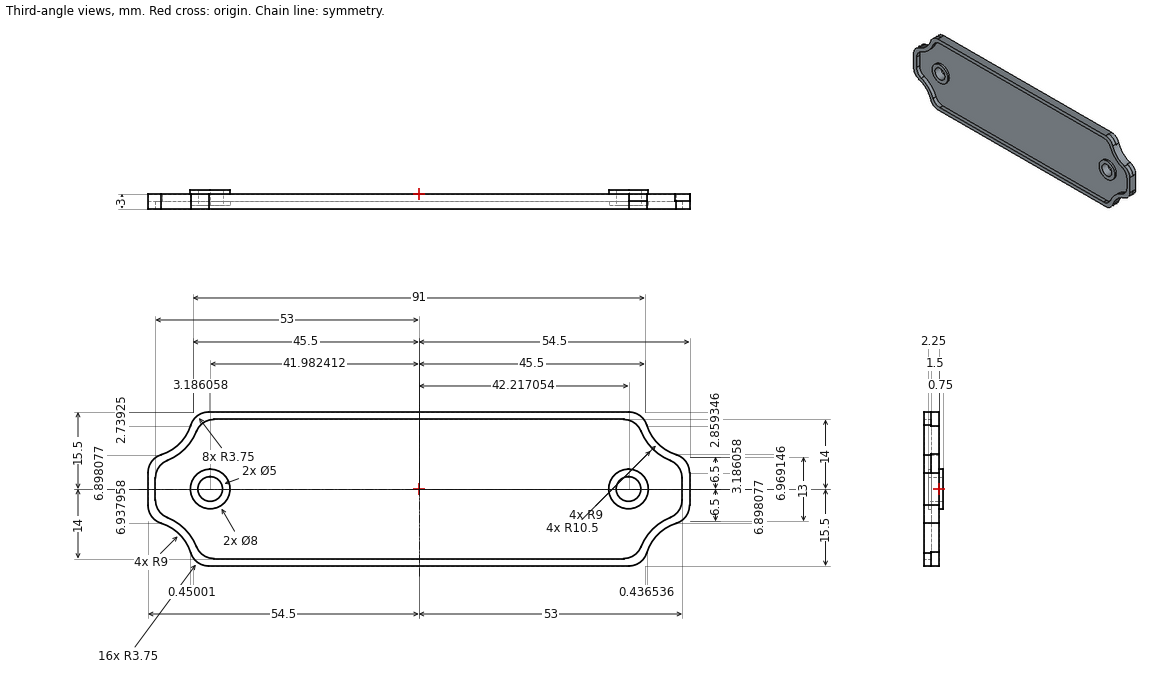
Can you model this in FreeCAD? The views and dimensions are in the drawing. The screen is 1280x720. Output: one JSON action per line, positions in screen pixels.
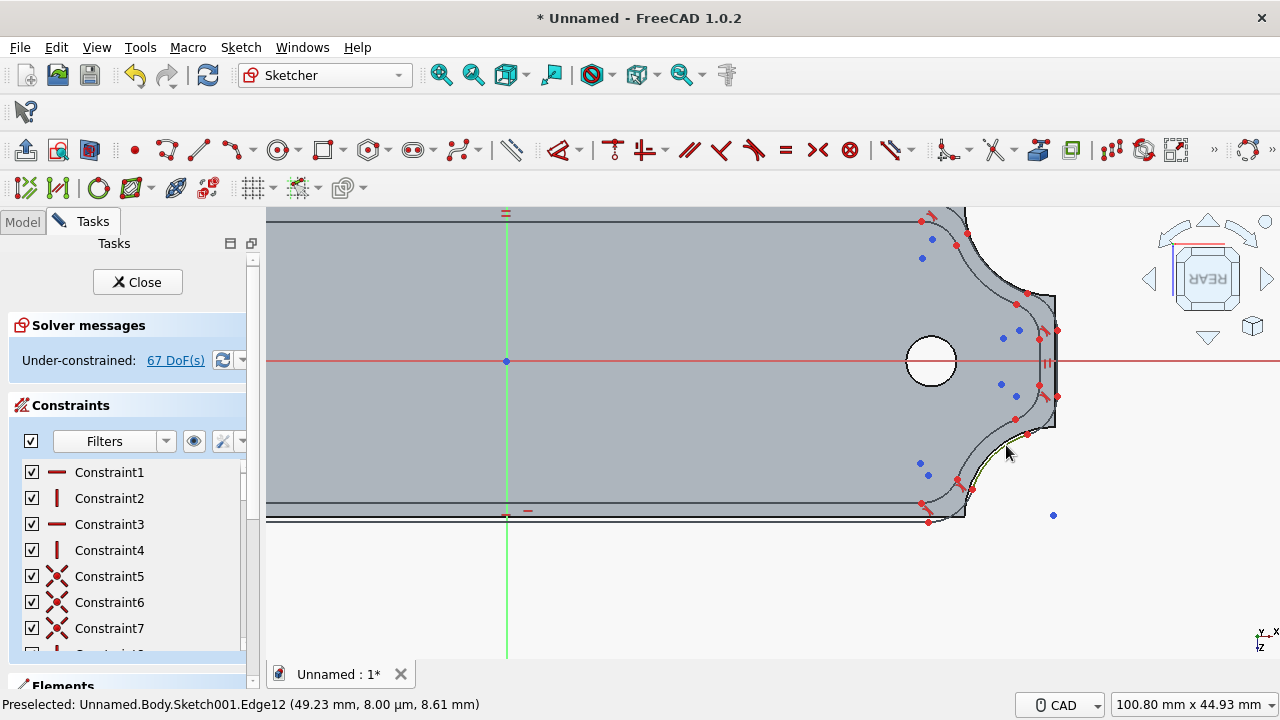
{"action": "left_click", "coordinate": [1042, 428]}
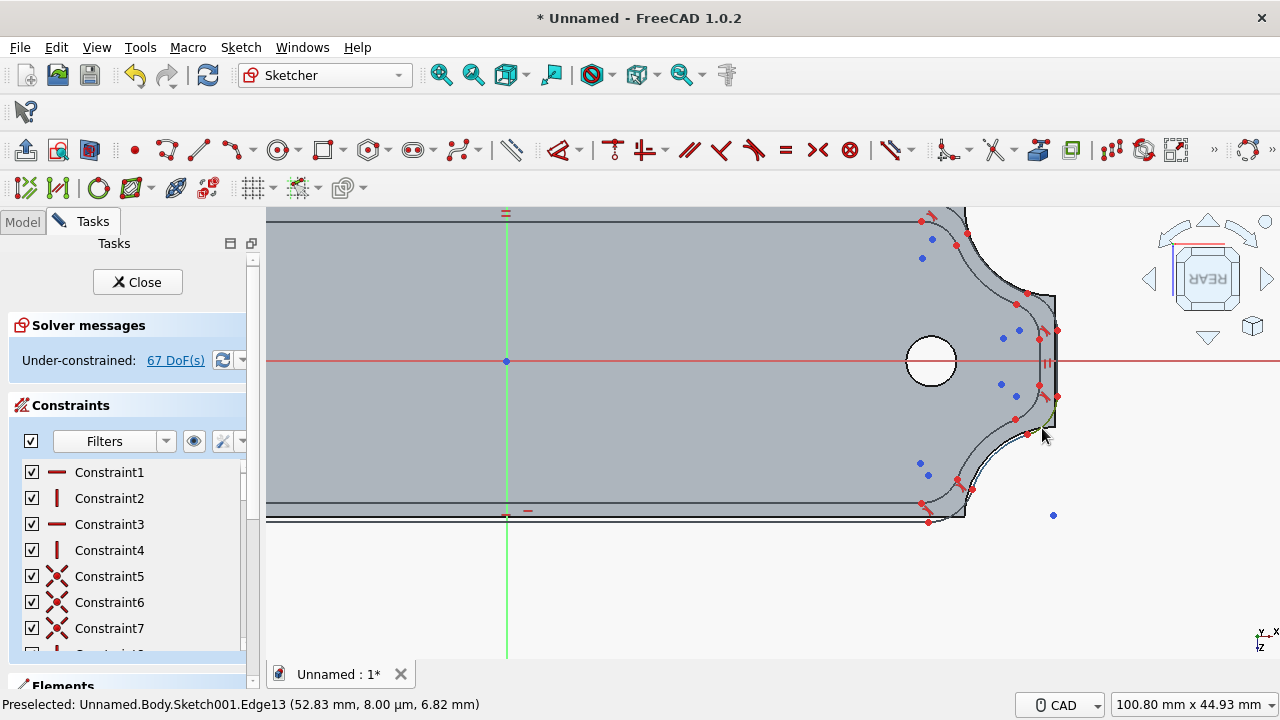
{"action": "left_click", "coordinate": [754, 150]}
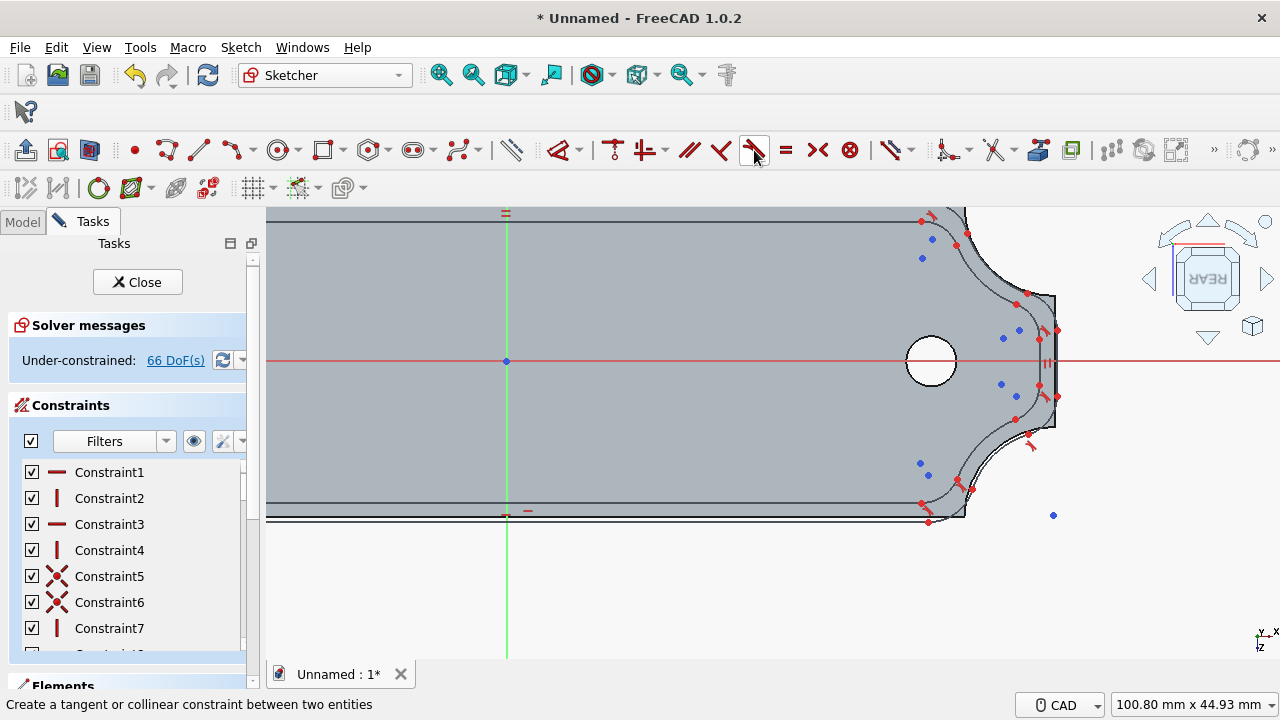
{"action": "left_click", "coordinate": [1054, 315]}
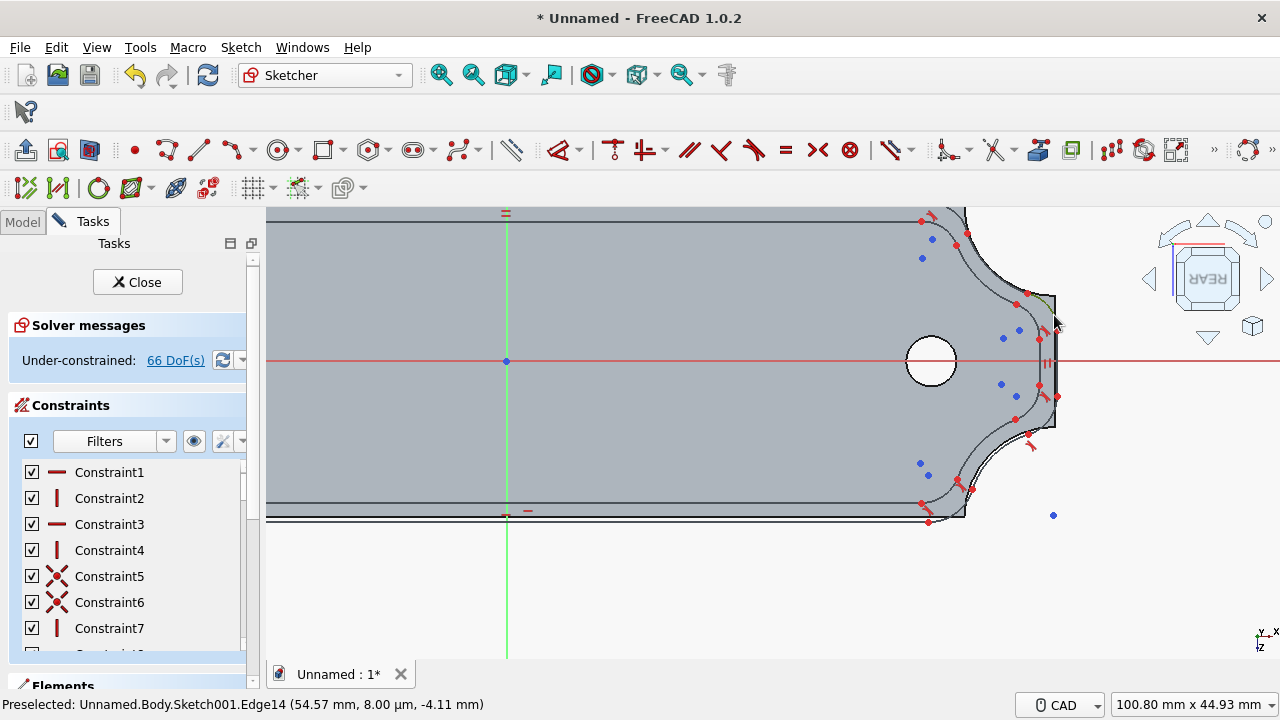
{"action": "left_click", "coordinate": [979, 257]}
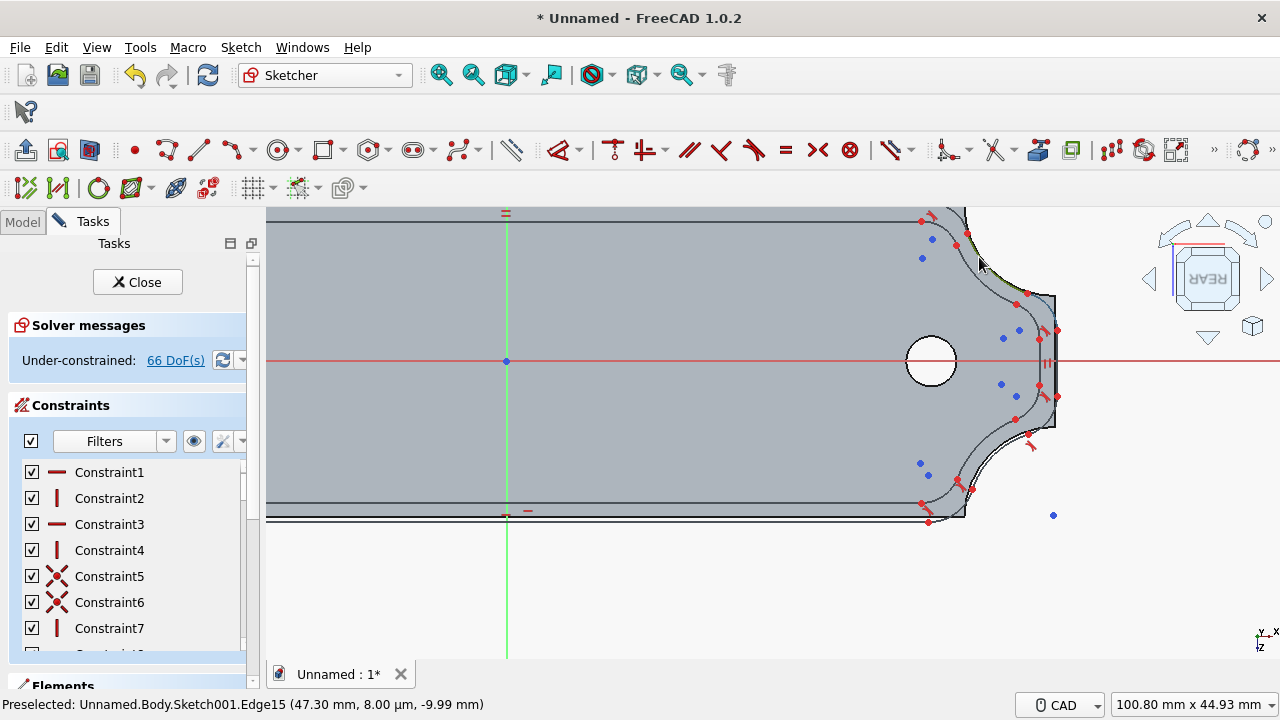
{"action": "left_click", "coordinate": [754, 150]}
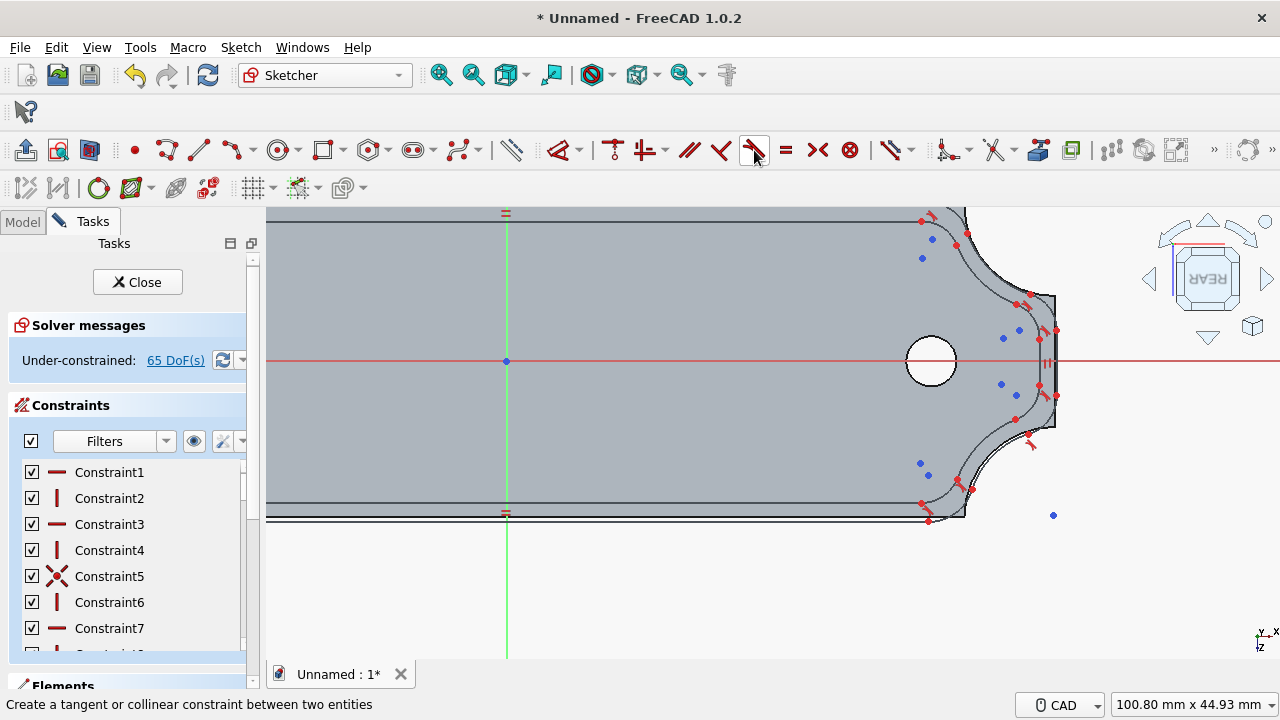
{"action": "left_click", "coordinate": [980, 257]}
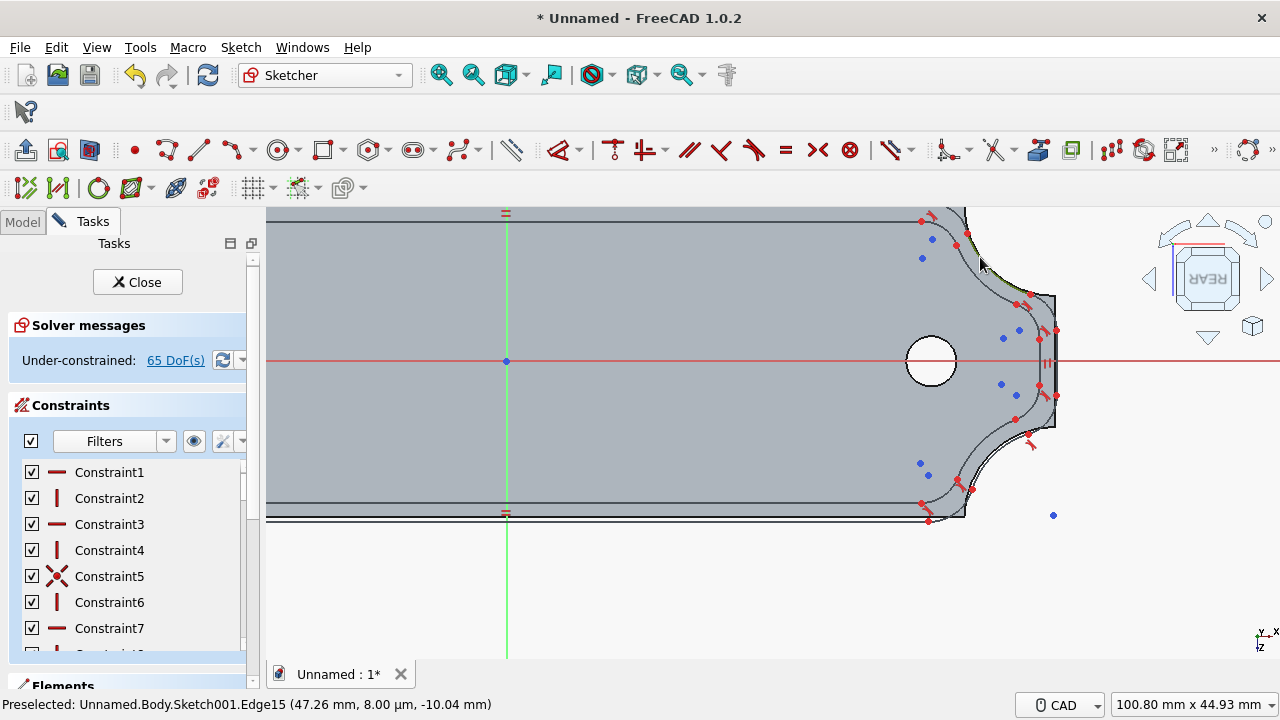
{"action": "scroll", "coordinate": [945, 520], "scroll_direction": "down", "scroll_amount": 3}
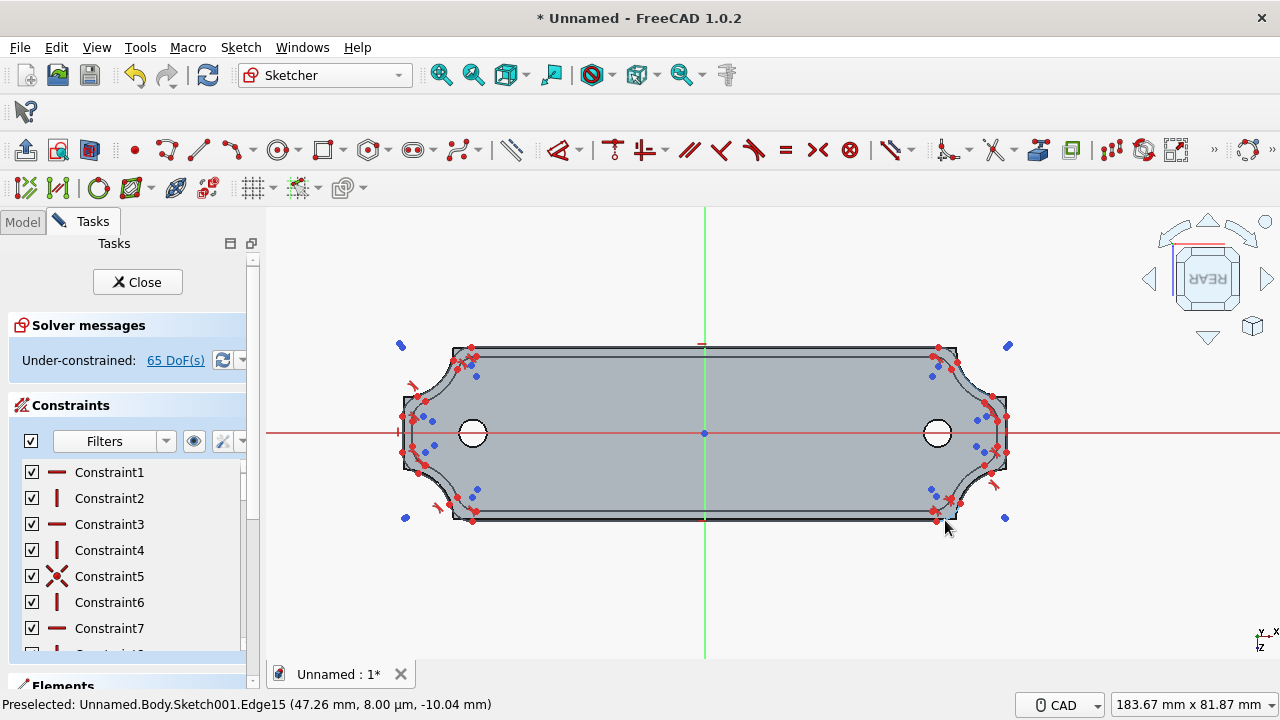
{"action": "scroll", "coordinate": [954, 356], "scroll_direction": "up", "scroll_amount": 3}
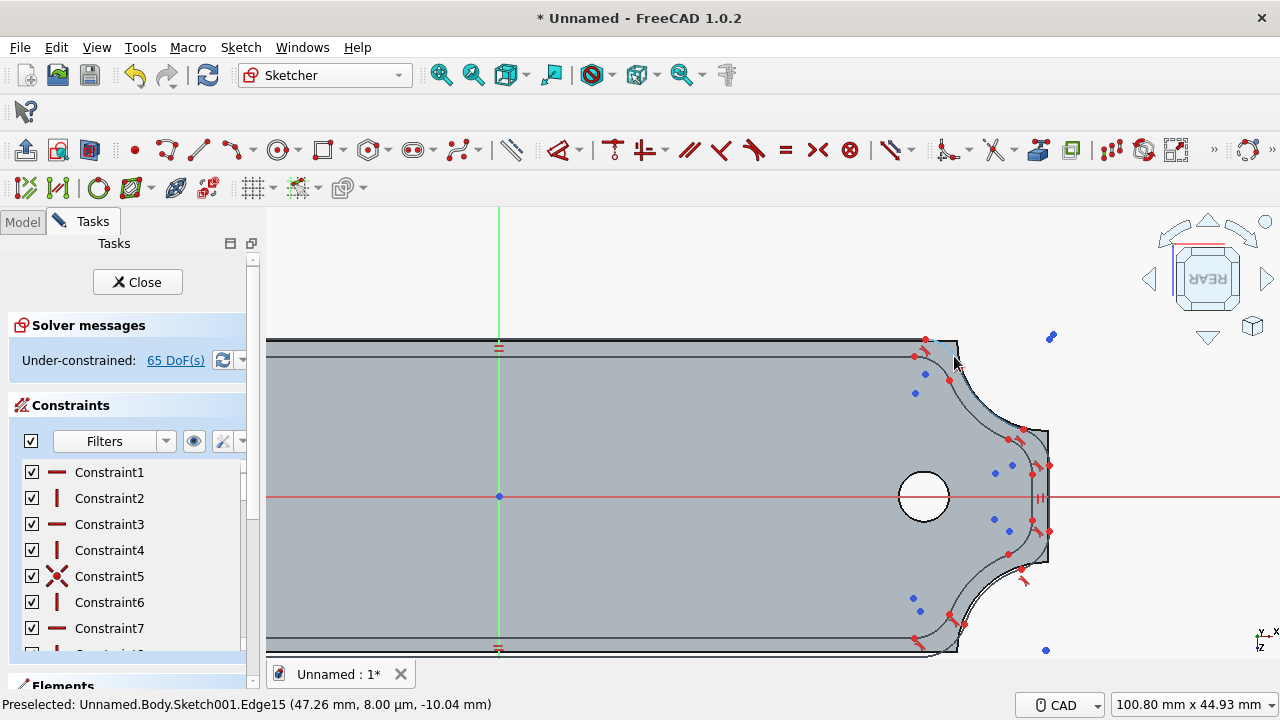
{"action": "left_click", "coordinate": [954, 355]}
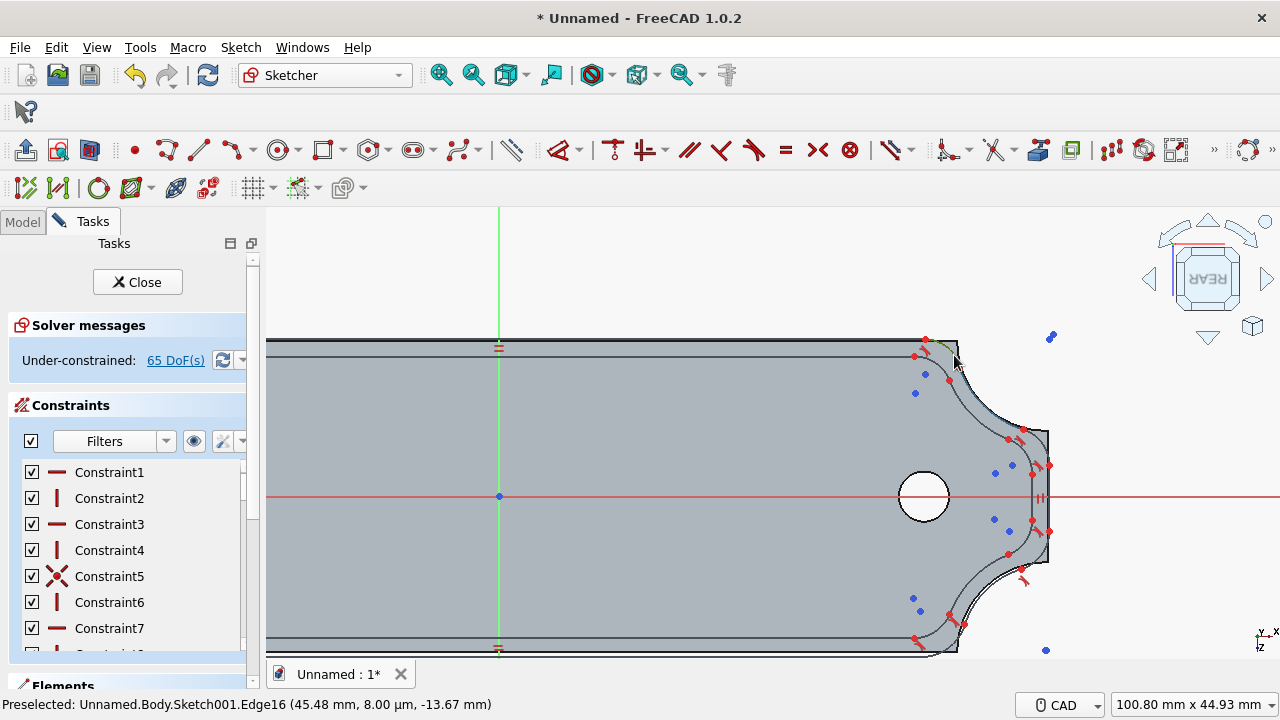
{"action": "left_click", "coordinate": [754, 150]}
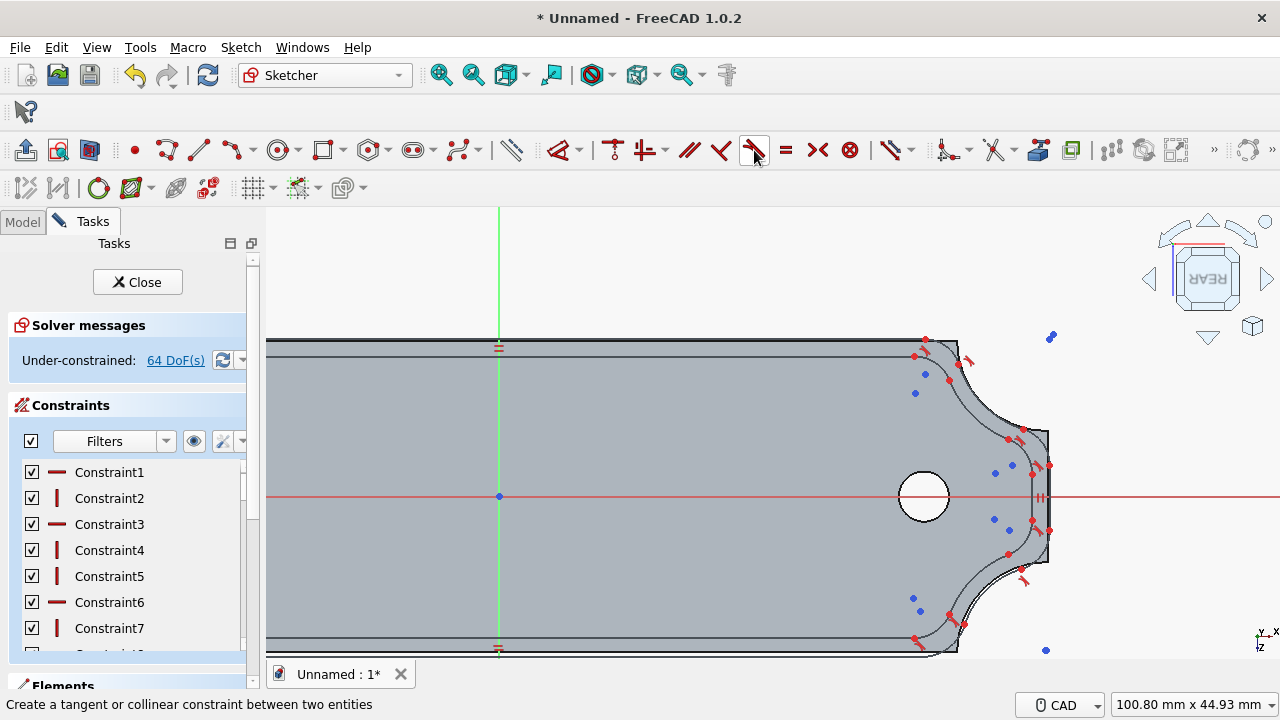
{"action": "scroll", "coordinate": [1032, 507], "scroll_direction": "up", "scroll_amount": 2}